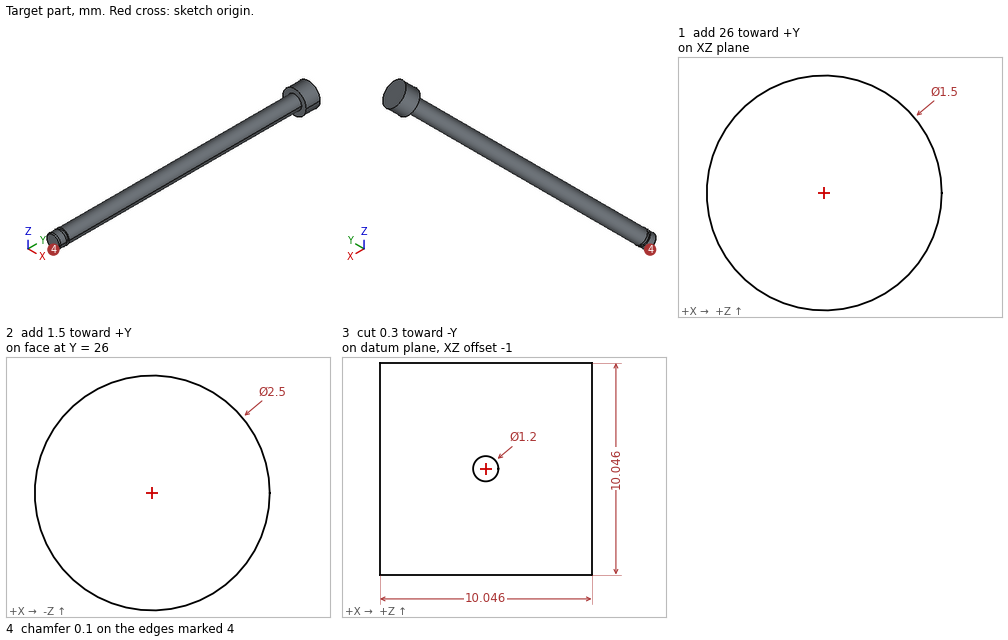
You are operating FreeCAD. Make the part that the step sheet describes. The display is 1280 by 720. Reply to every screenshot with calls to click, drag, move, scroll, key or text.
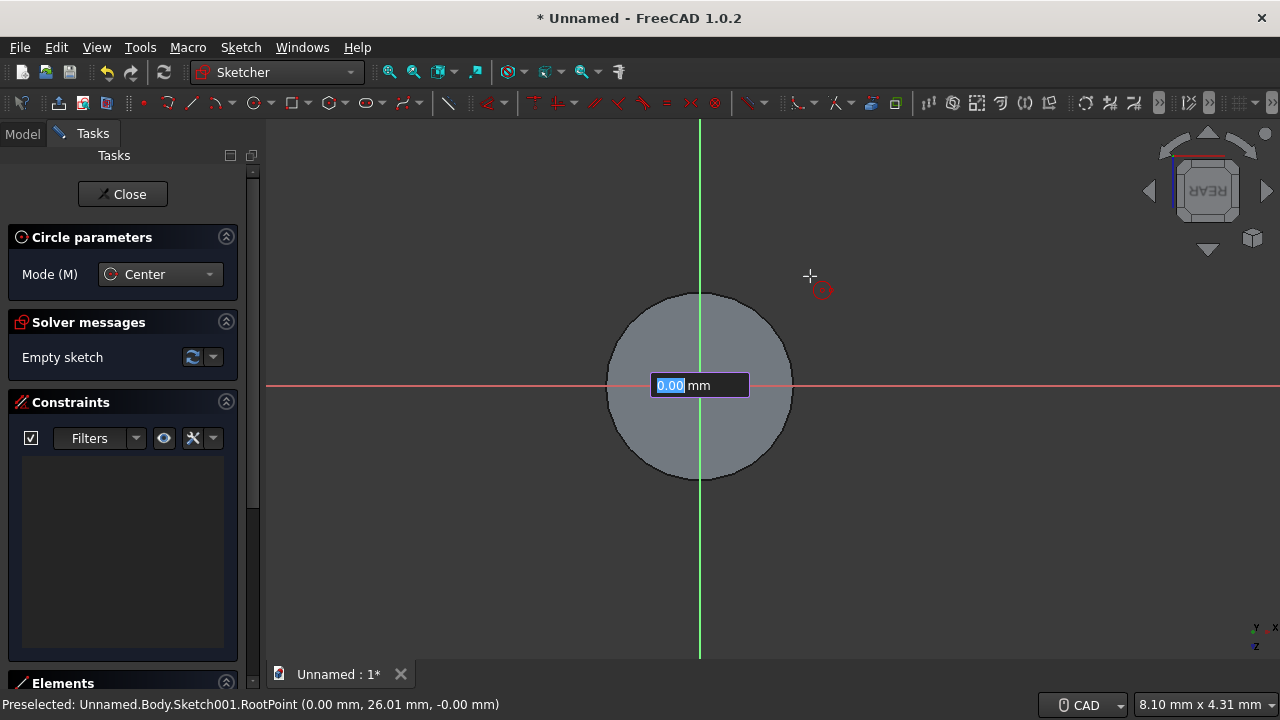
text(2.5)
key(Return)
key(Escape)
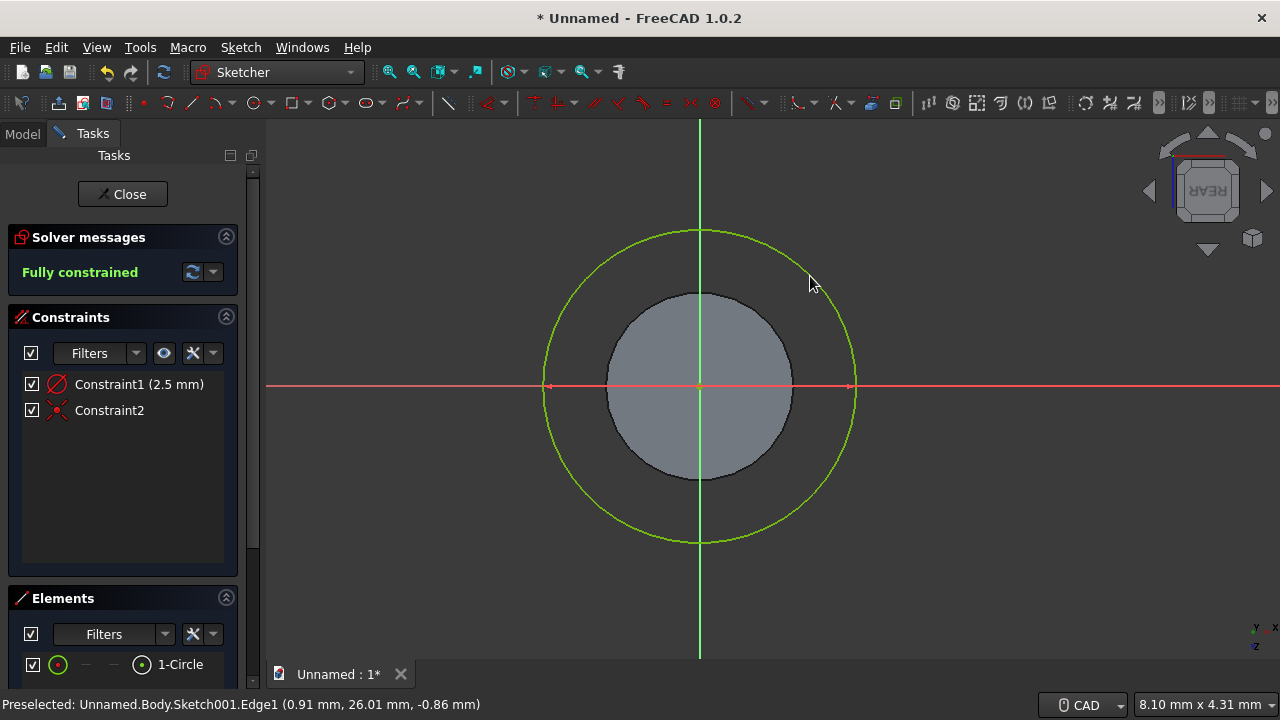
click(123, 194)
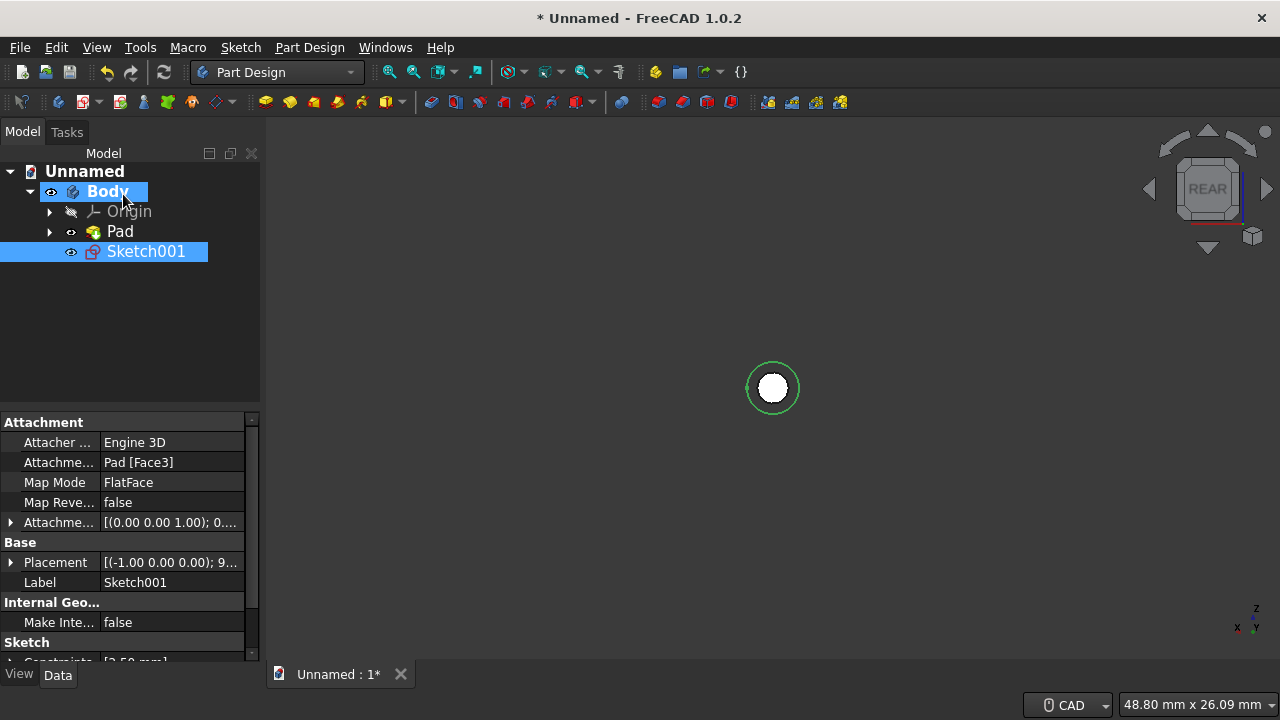
click(266, 102)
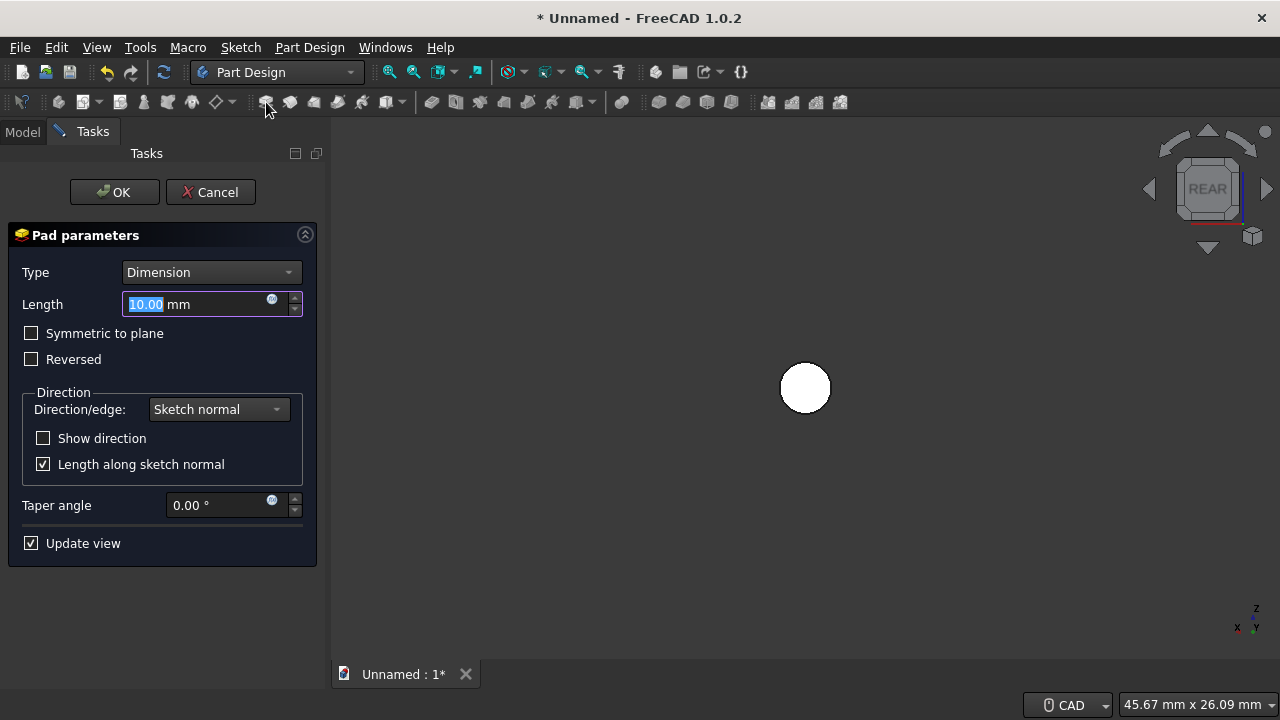
text(1.5)
key(Tab)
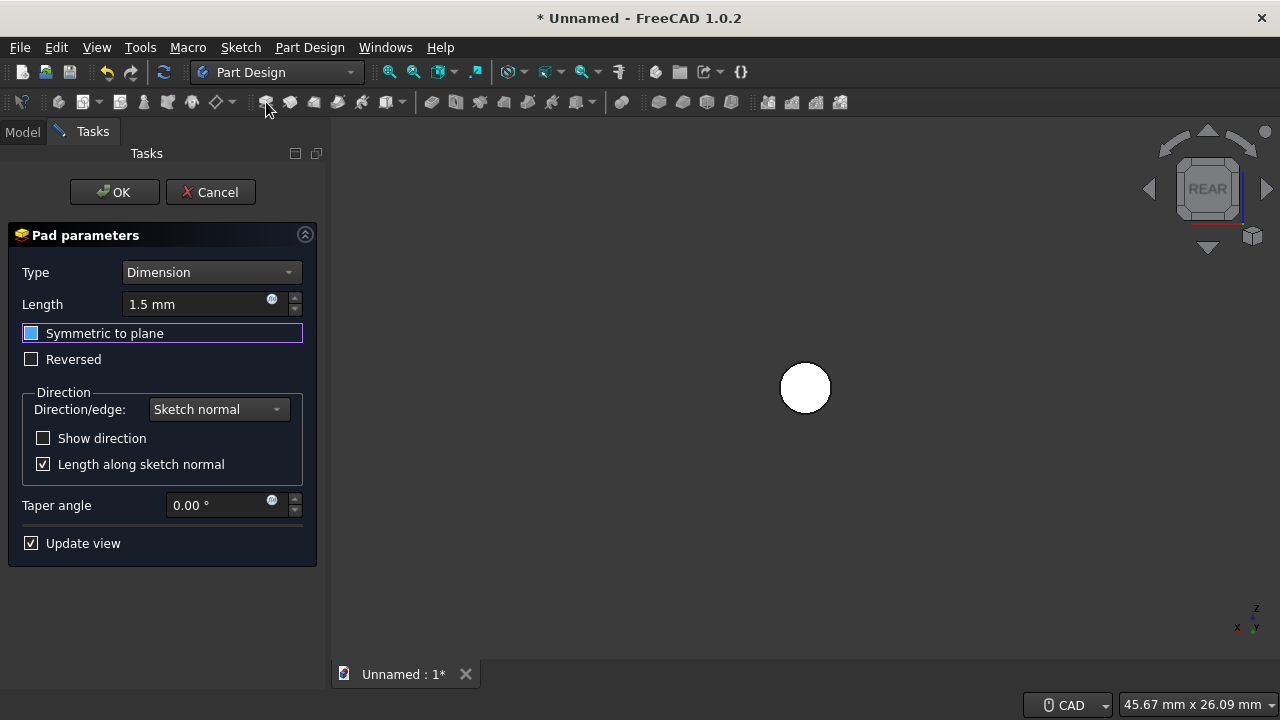
click(115, 192)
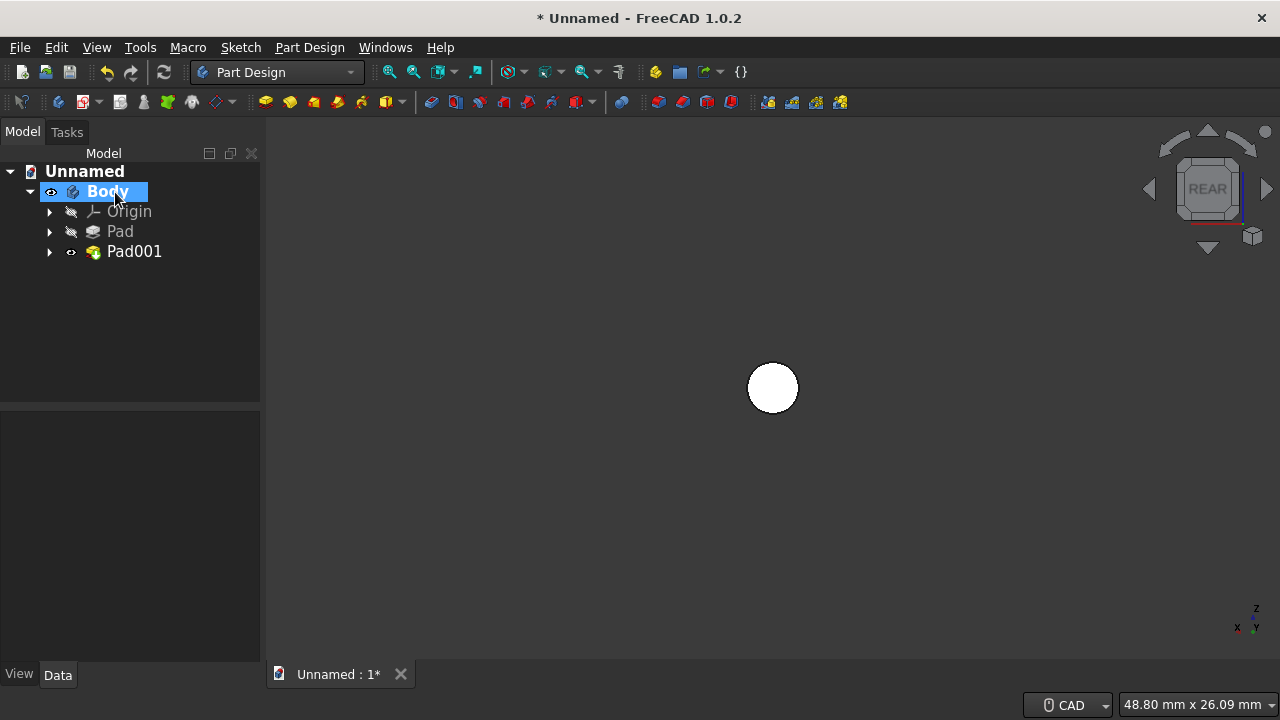
click(390, 72)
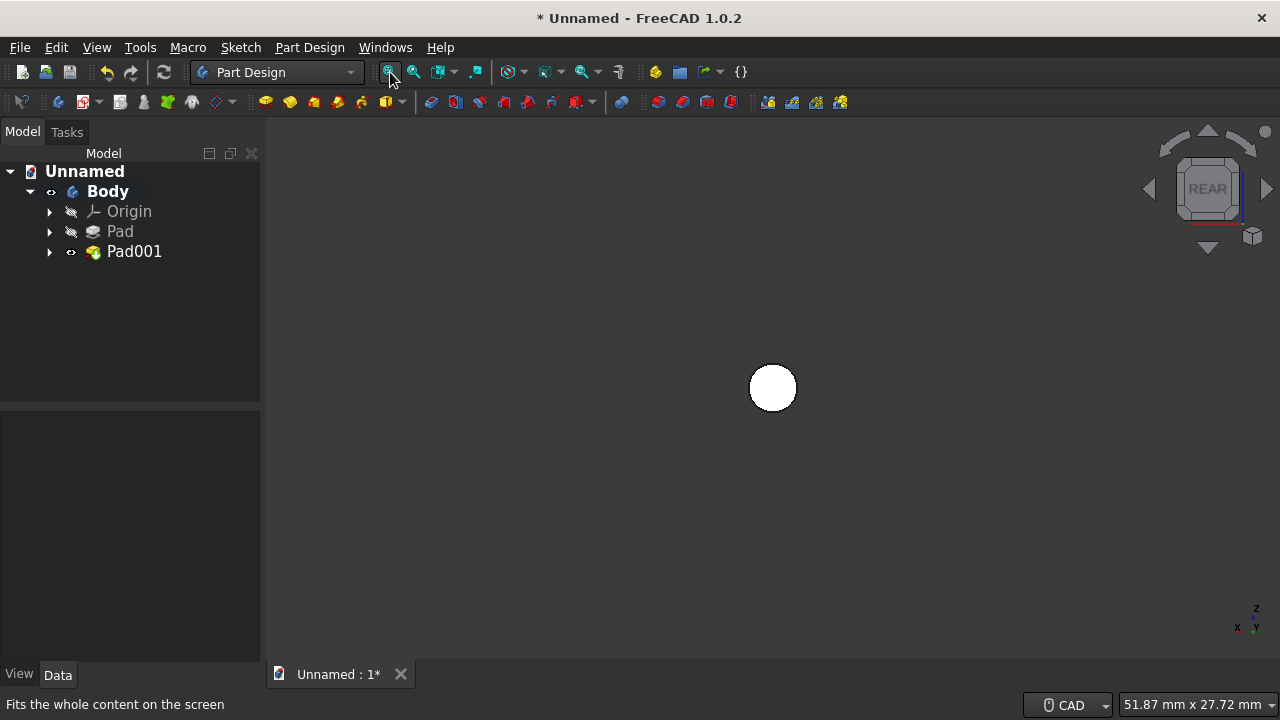
click(50, 212)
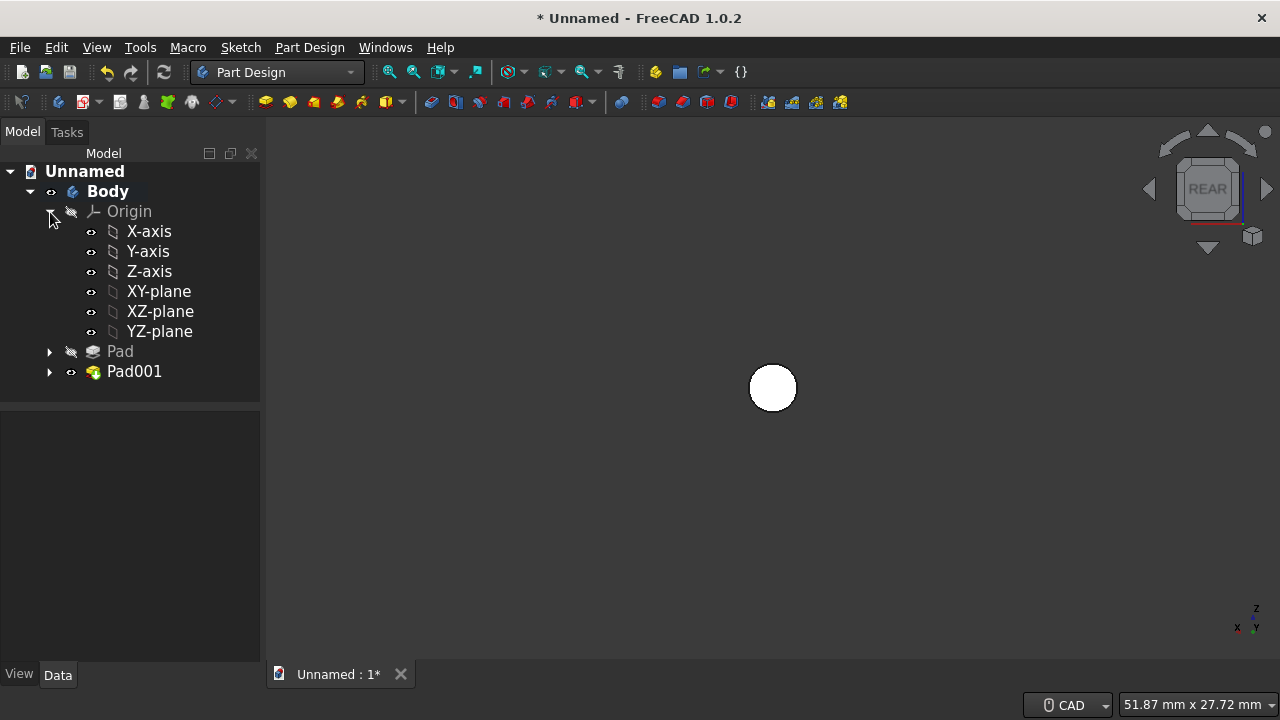
click(136, 312)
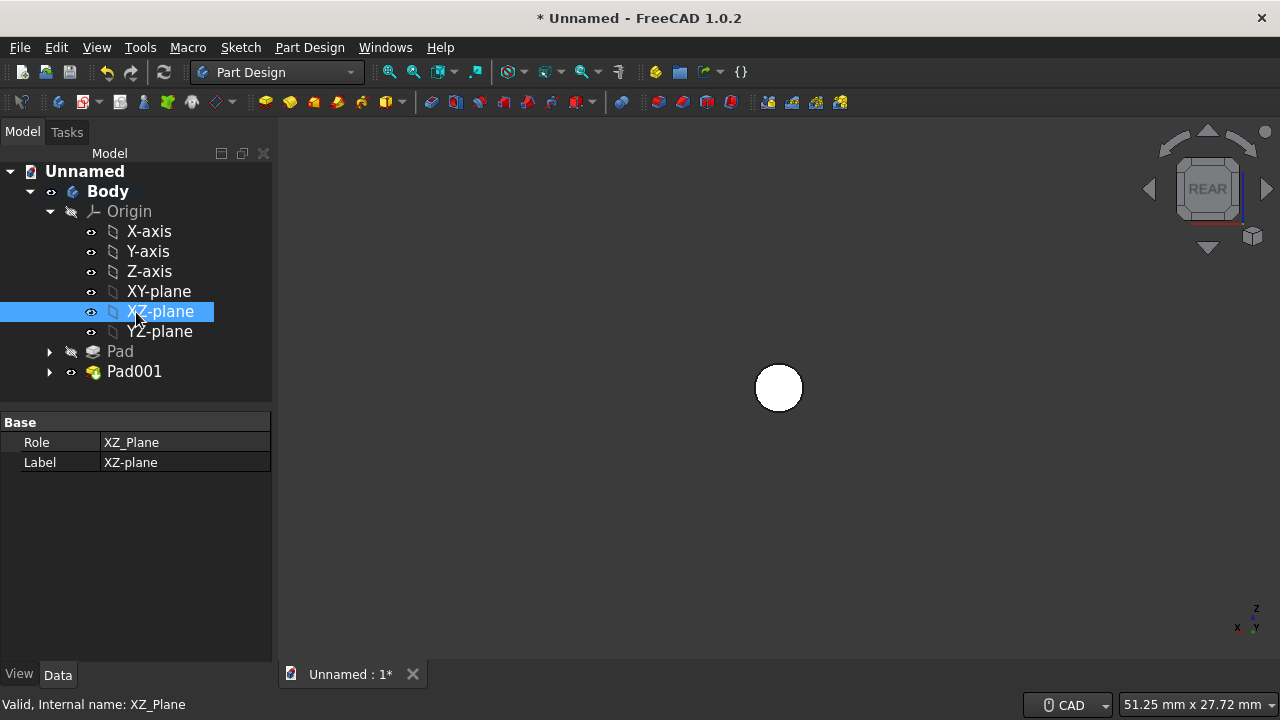
click(216, 102)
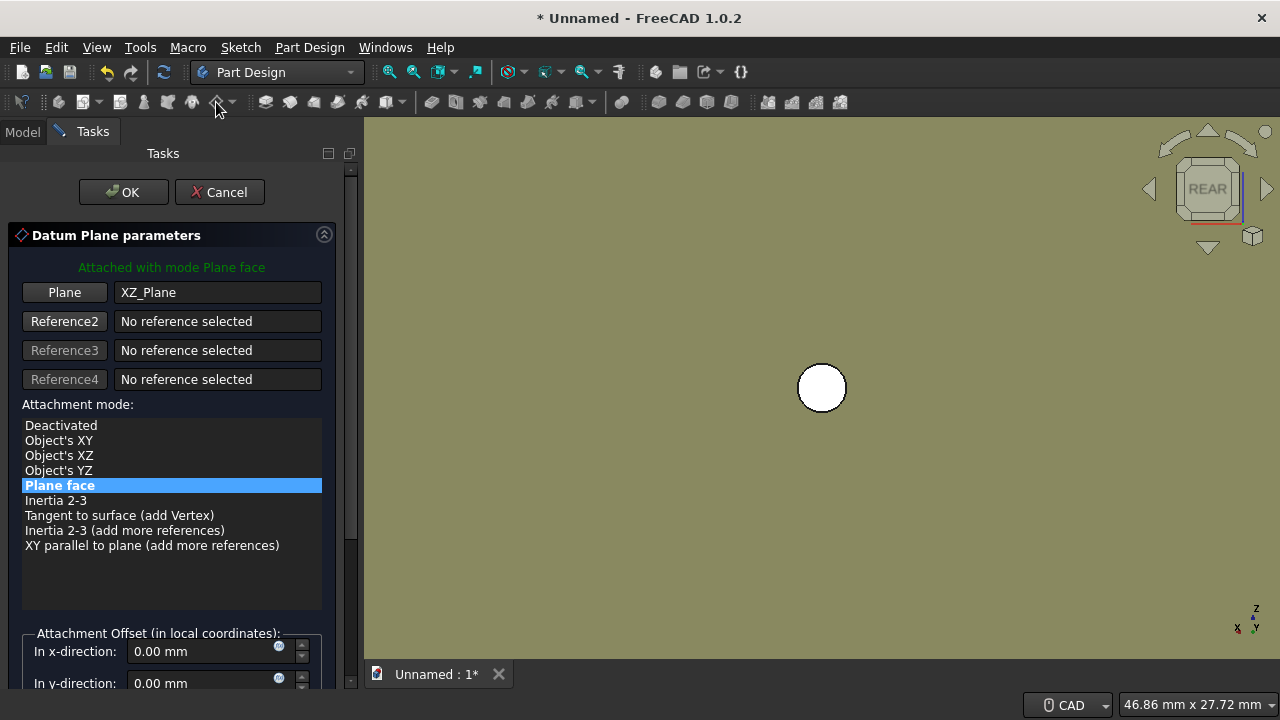
scroll(351, 426, down, 2)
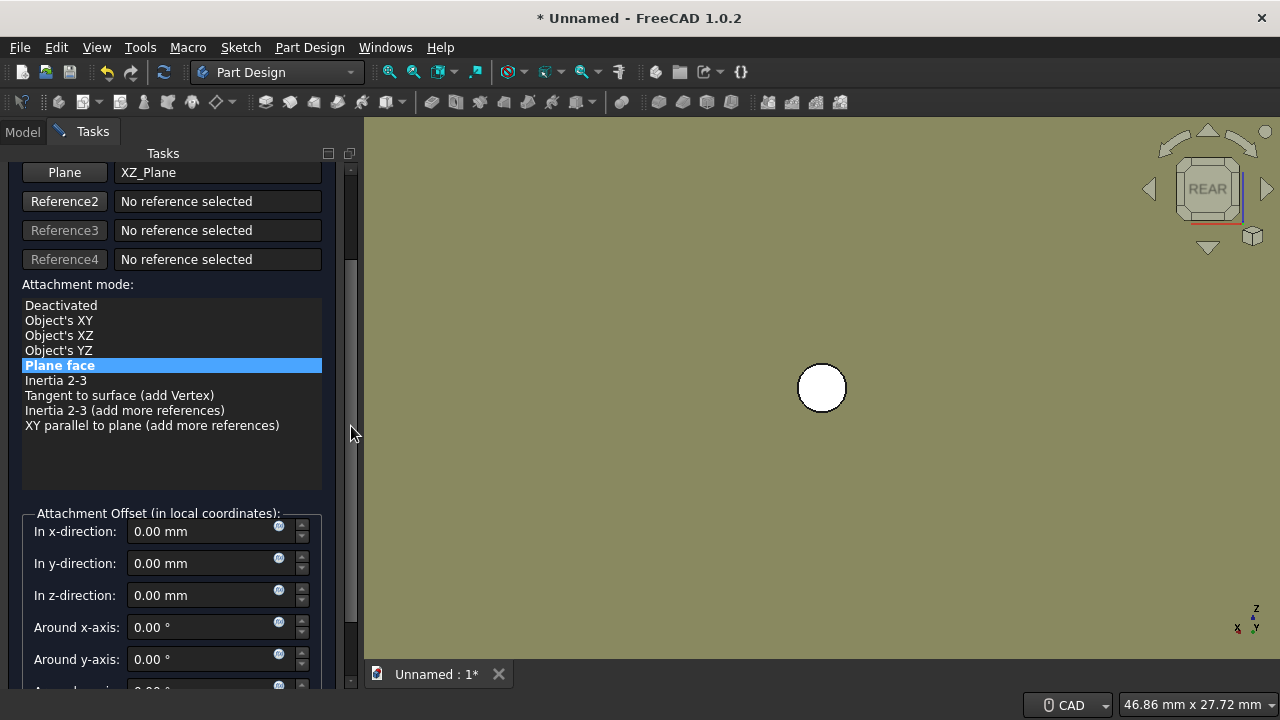
triple_click(210, 595)